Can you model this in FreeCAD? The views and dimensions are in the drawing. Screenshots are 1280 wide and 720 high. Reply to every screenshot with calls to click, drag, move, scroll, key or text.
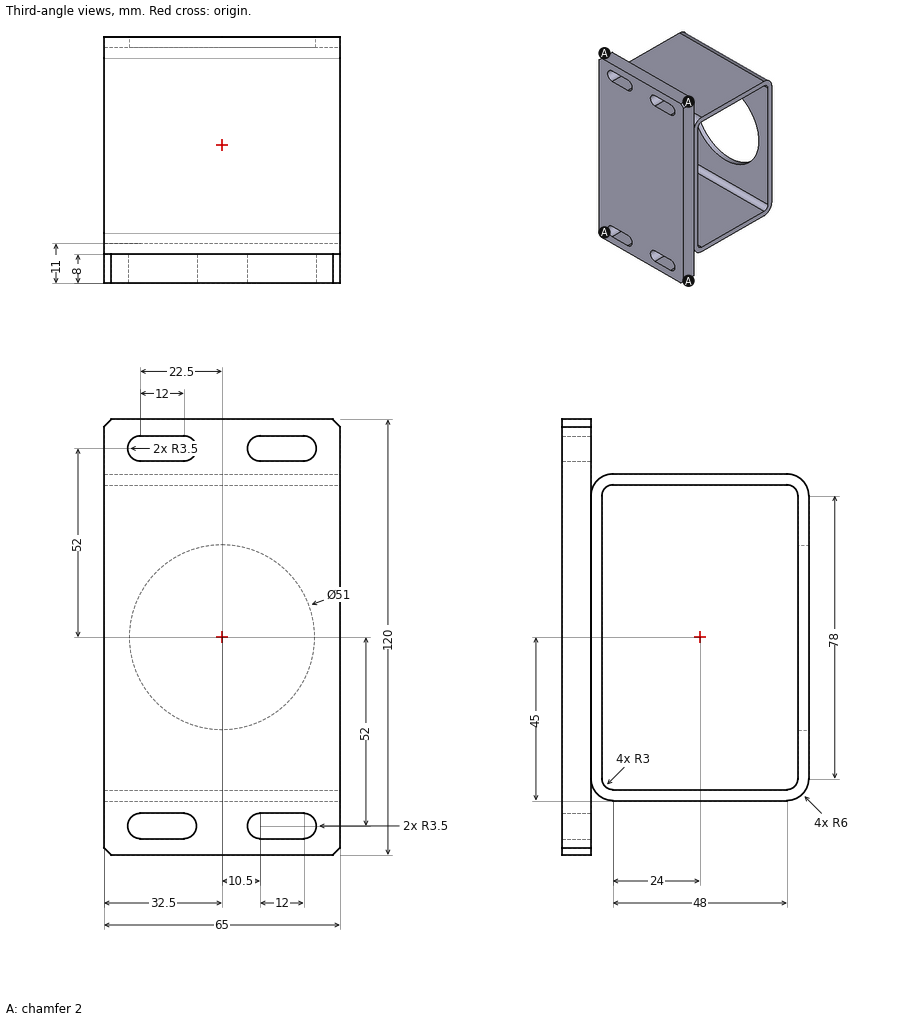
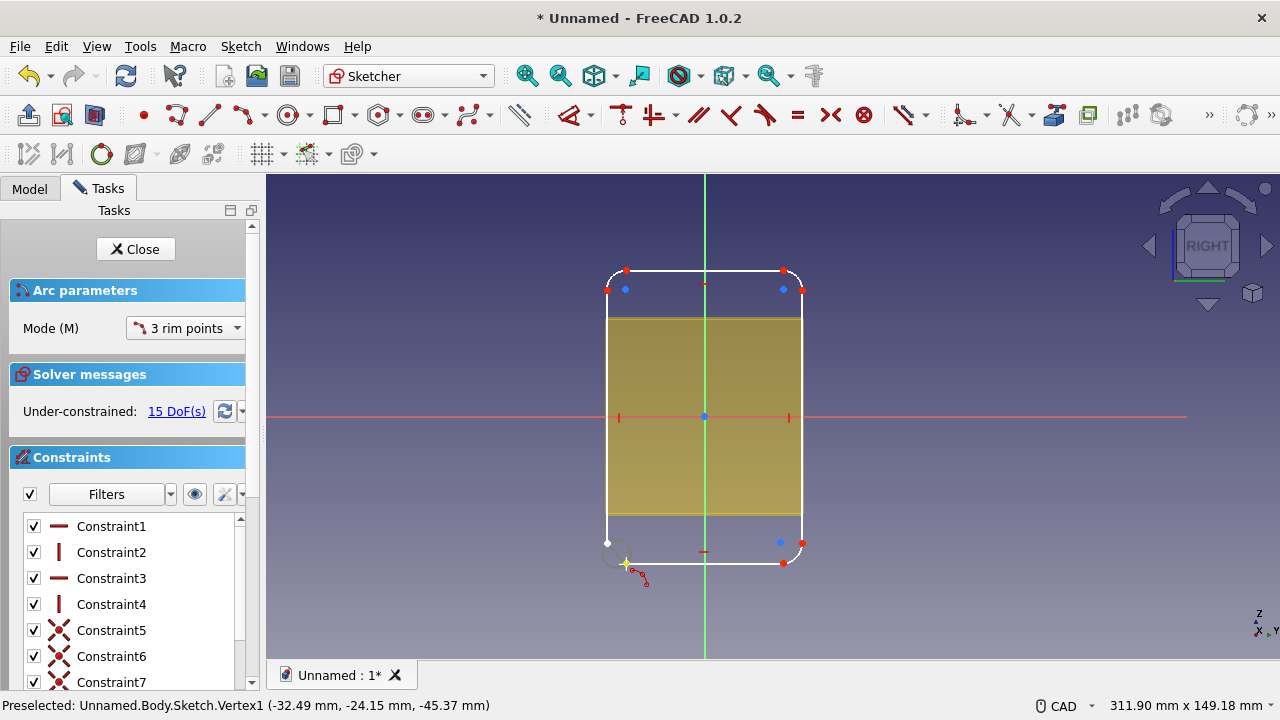
scroll(613, 557, up, 6)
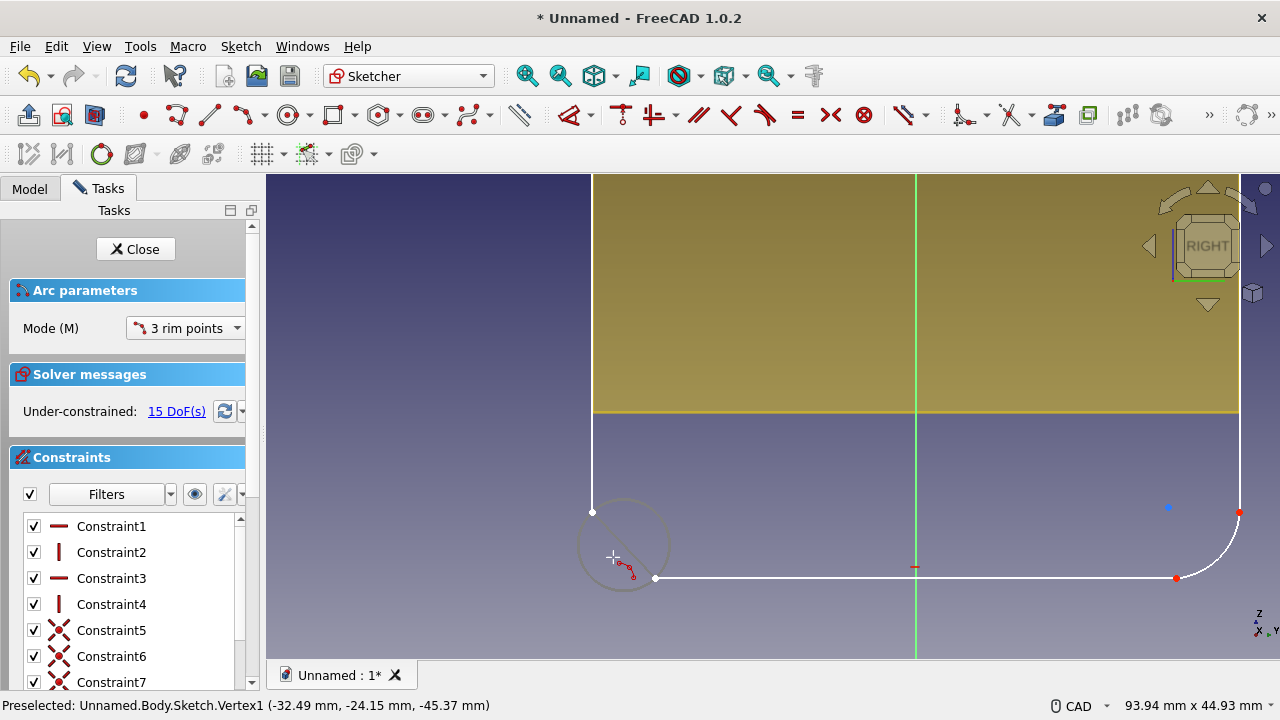
click(611, 555)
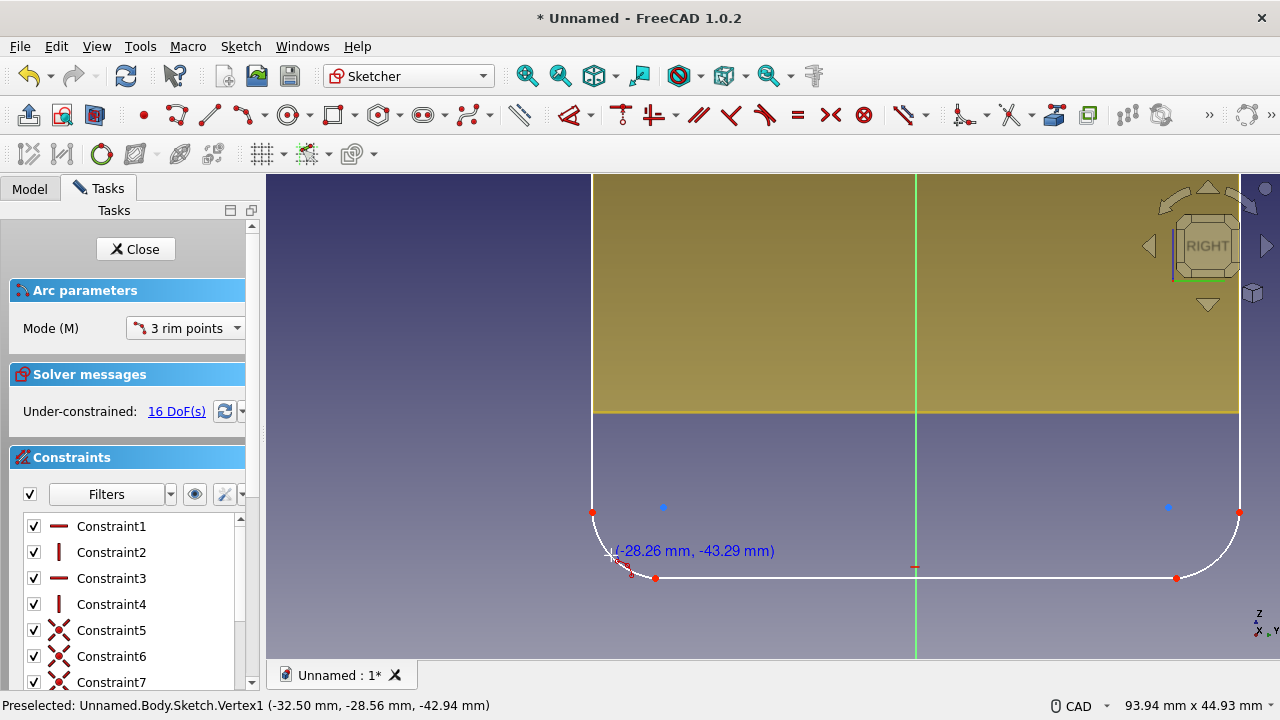
click(210, 116)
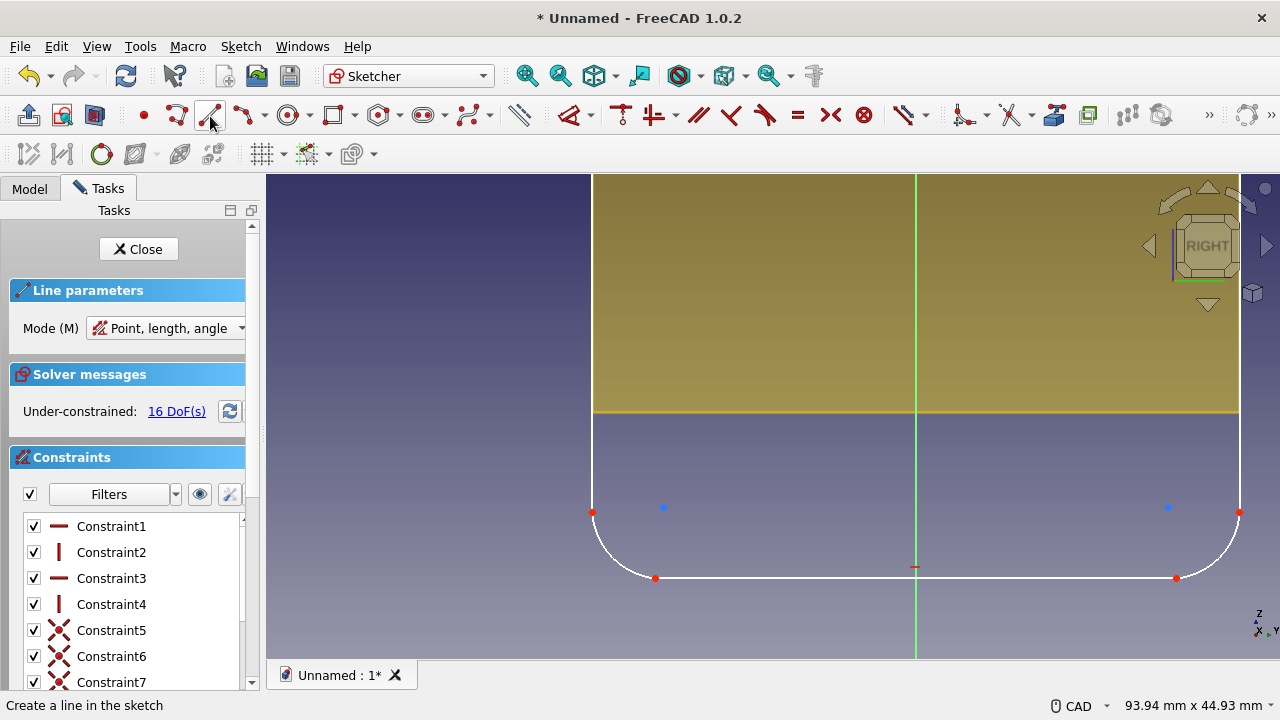
scroll(613, 558, down, 6)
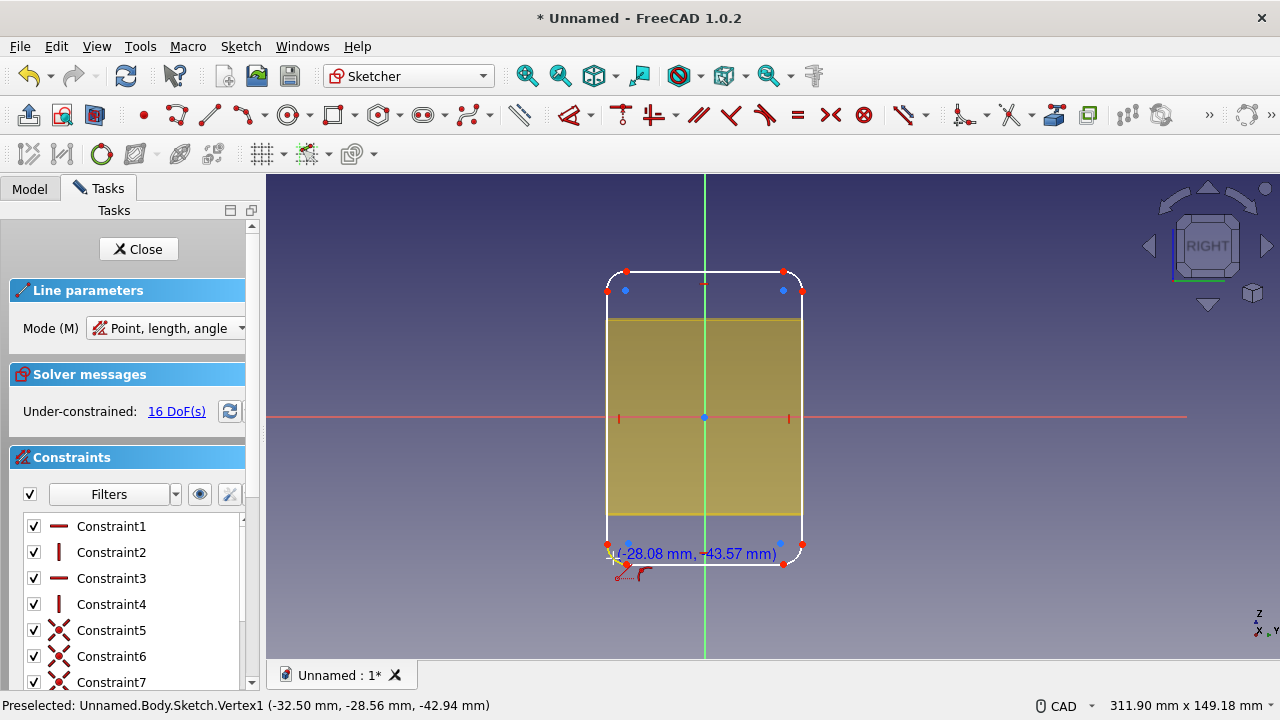
scroll(783, 554, up, 3)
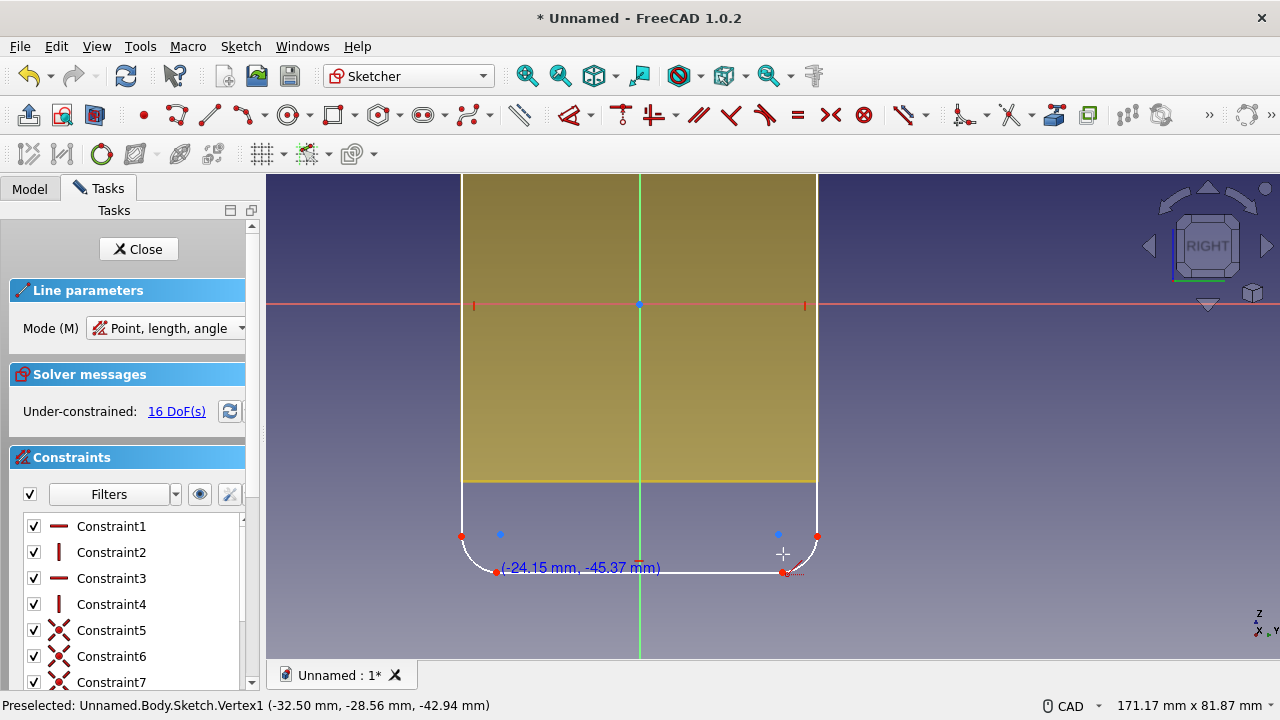
click(782, 553)
click(497, 553)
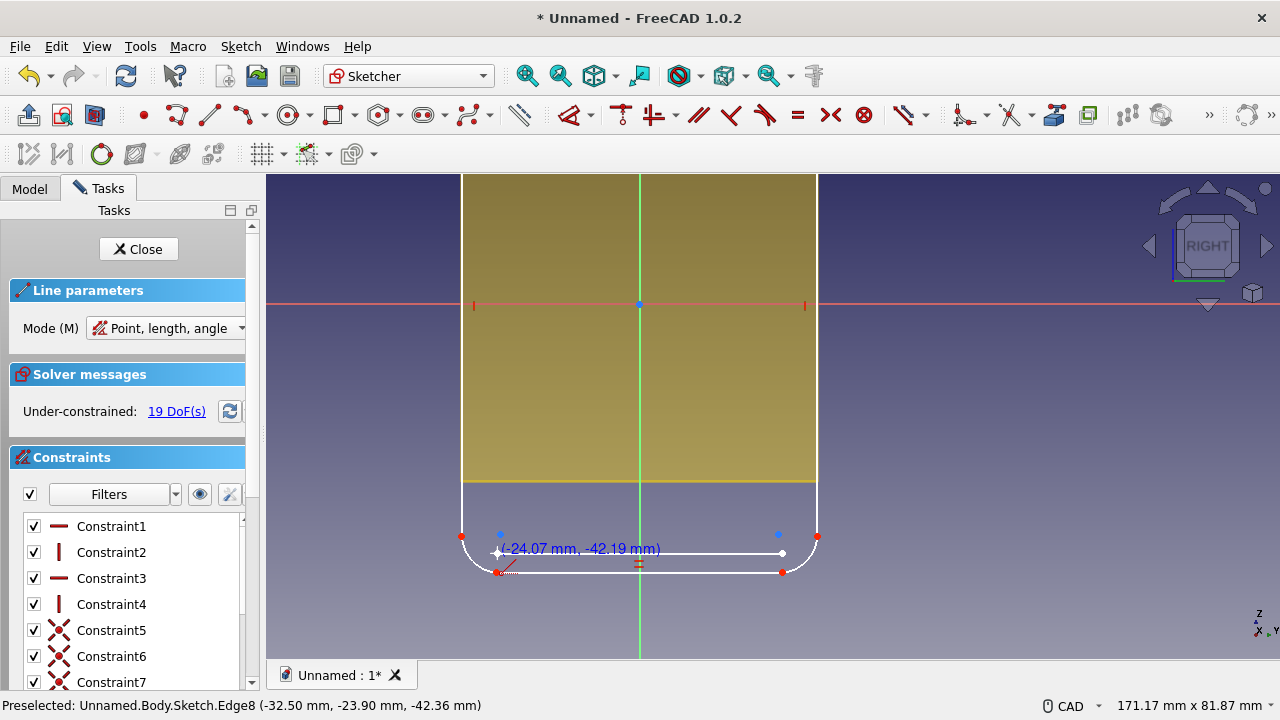
click(480, 535)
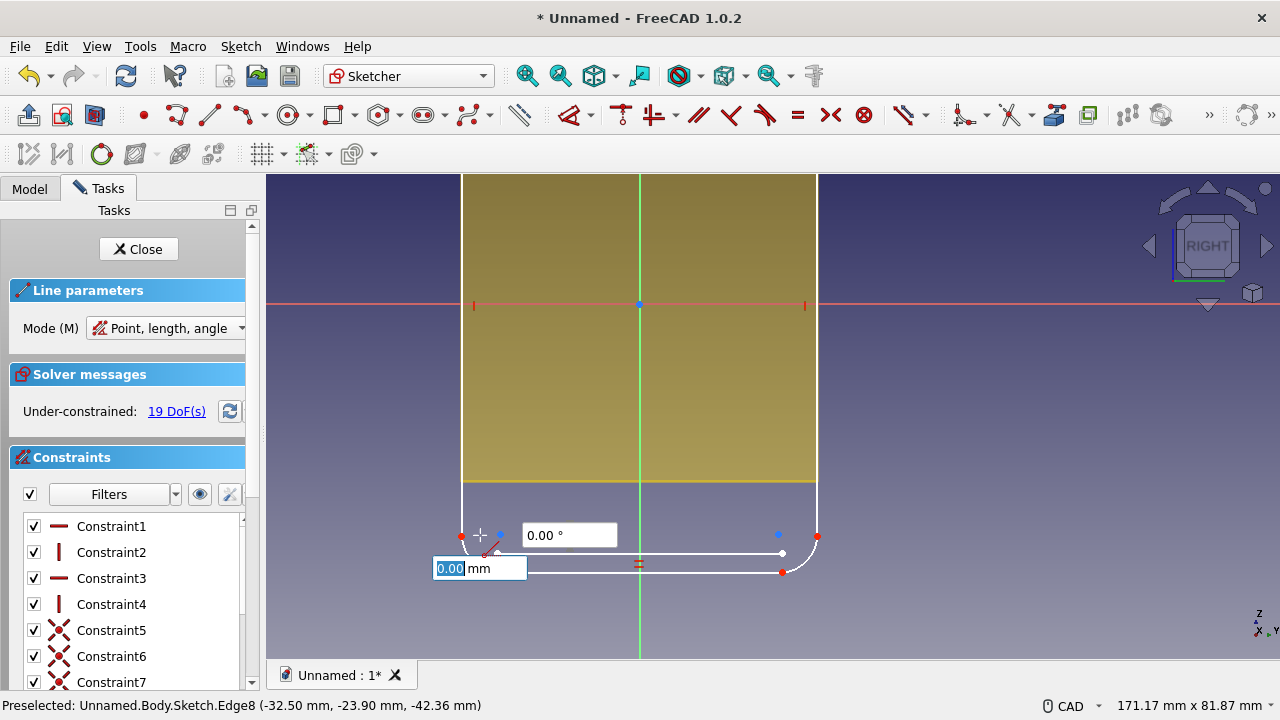
scroll(783, 553, down, 3)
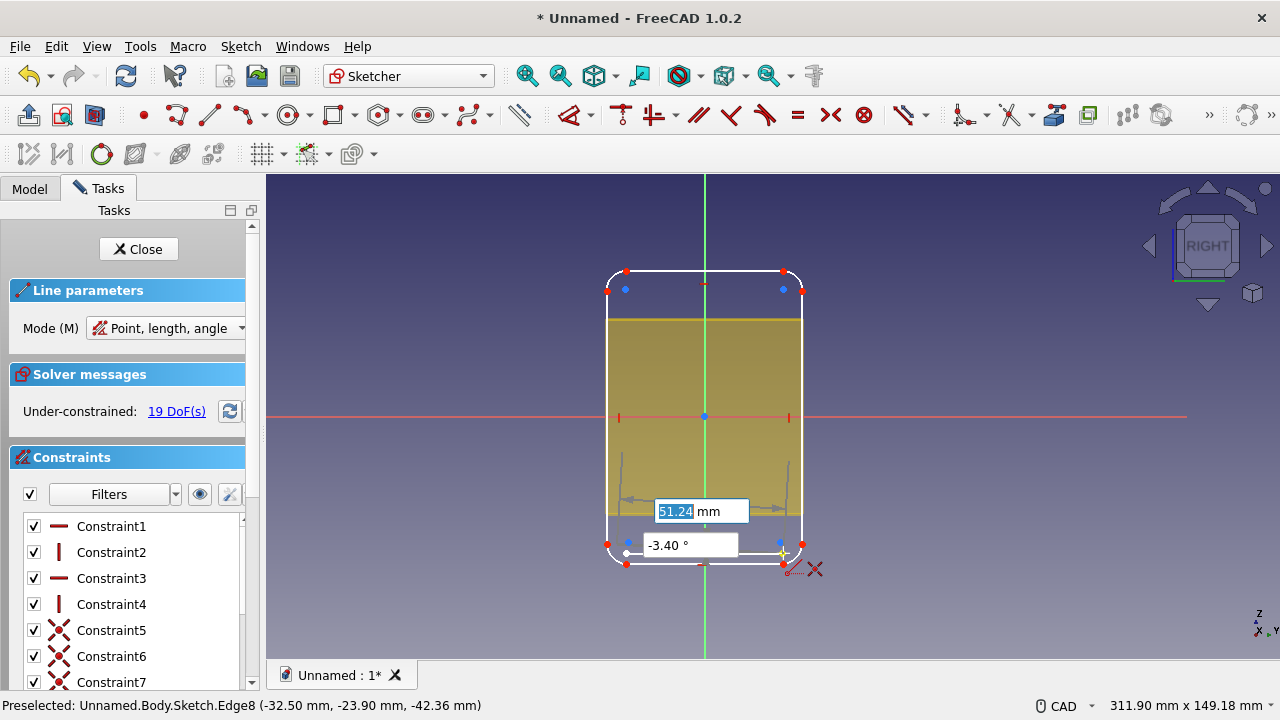
scroll(617, 290, up, 3)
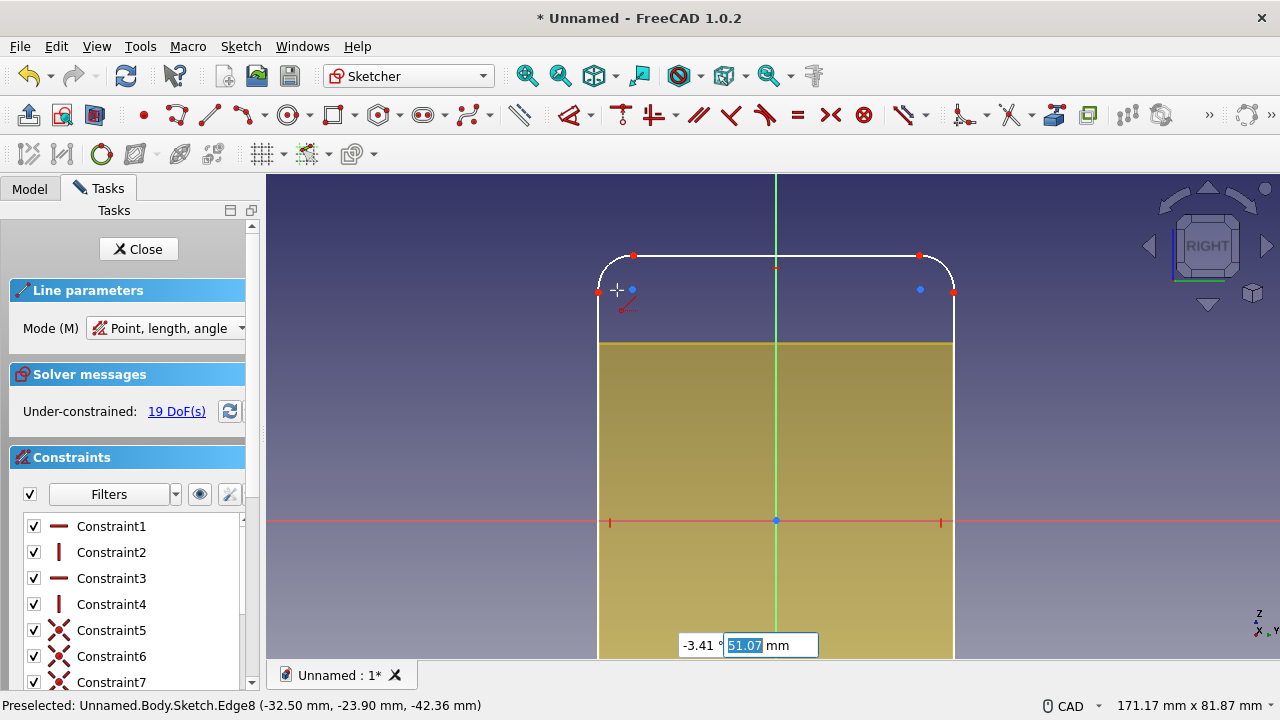
click(617, 290)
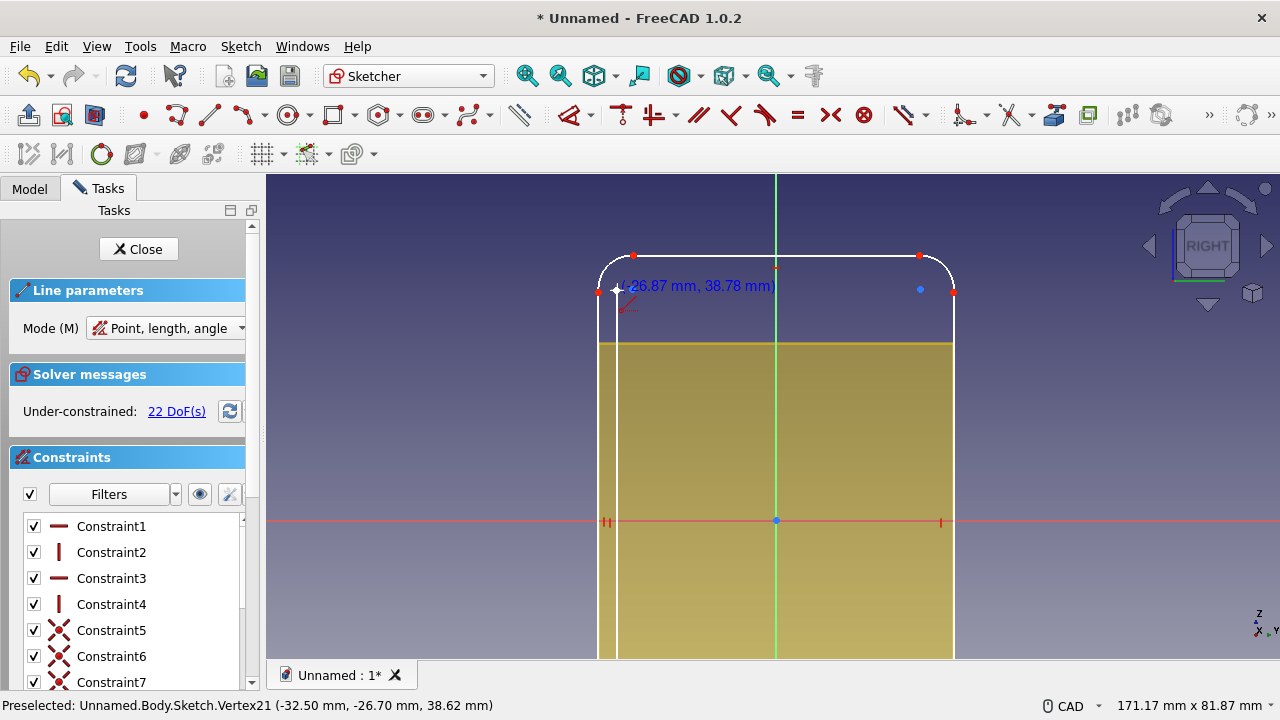
click(634, 272)
click(918, 272)